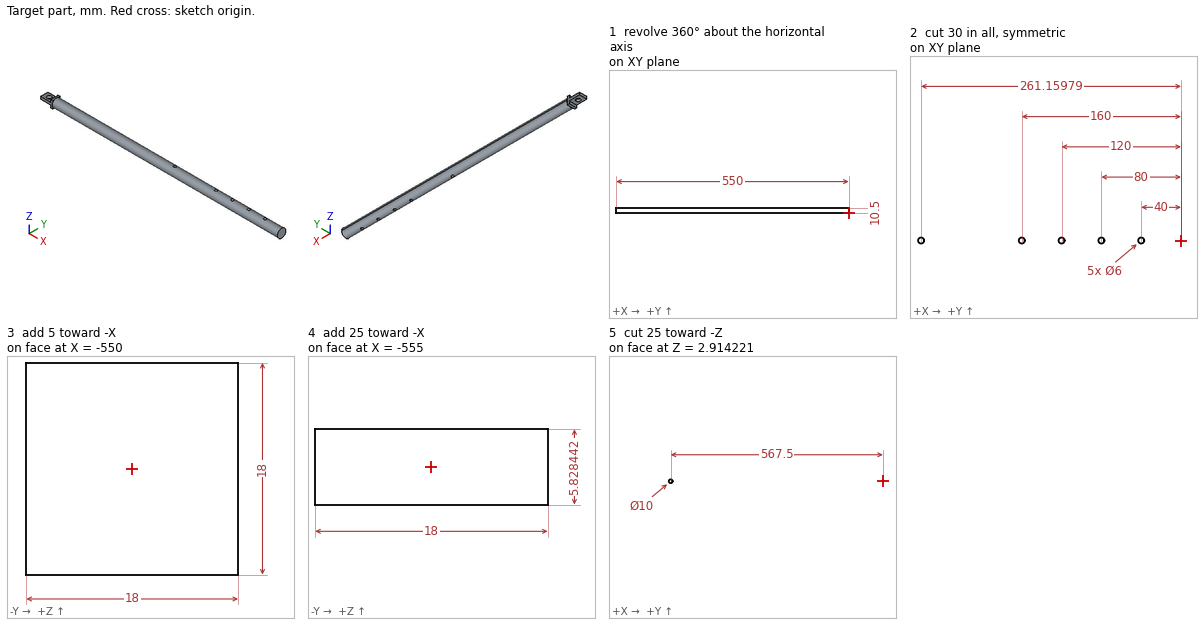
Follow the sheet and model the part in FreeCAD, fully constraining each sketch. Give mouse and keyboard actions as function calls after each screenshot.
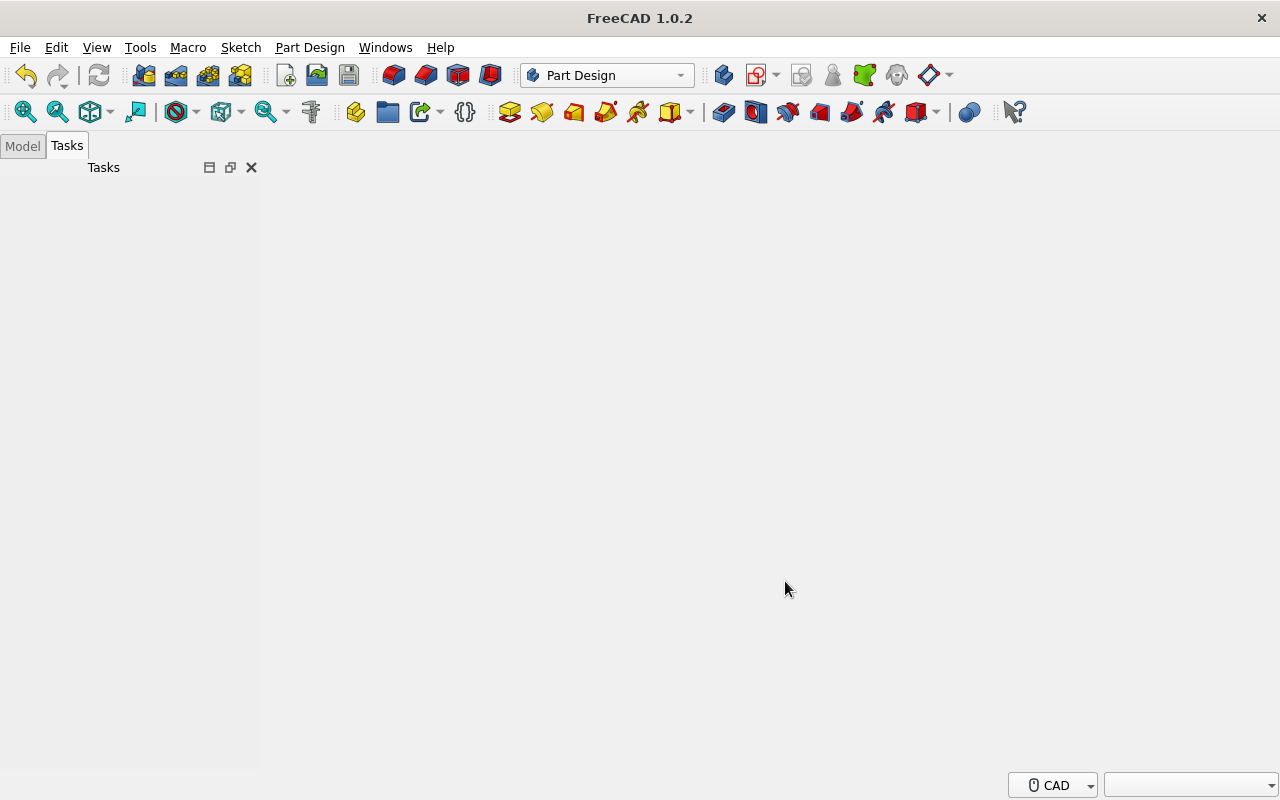
click(286, 76)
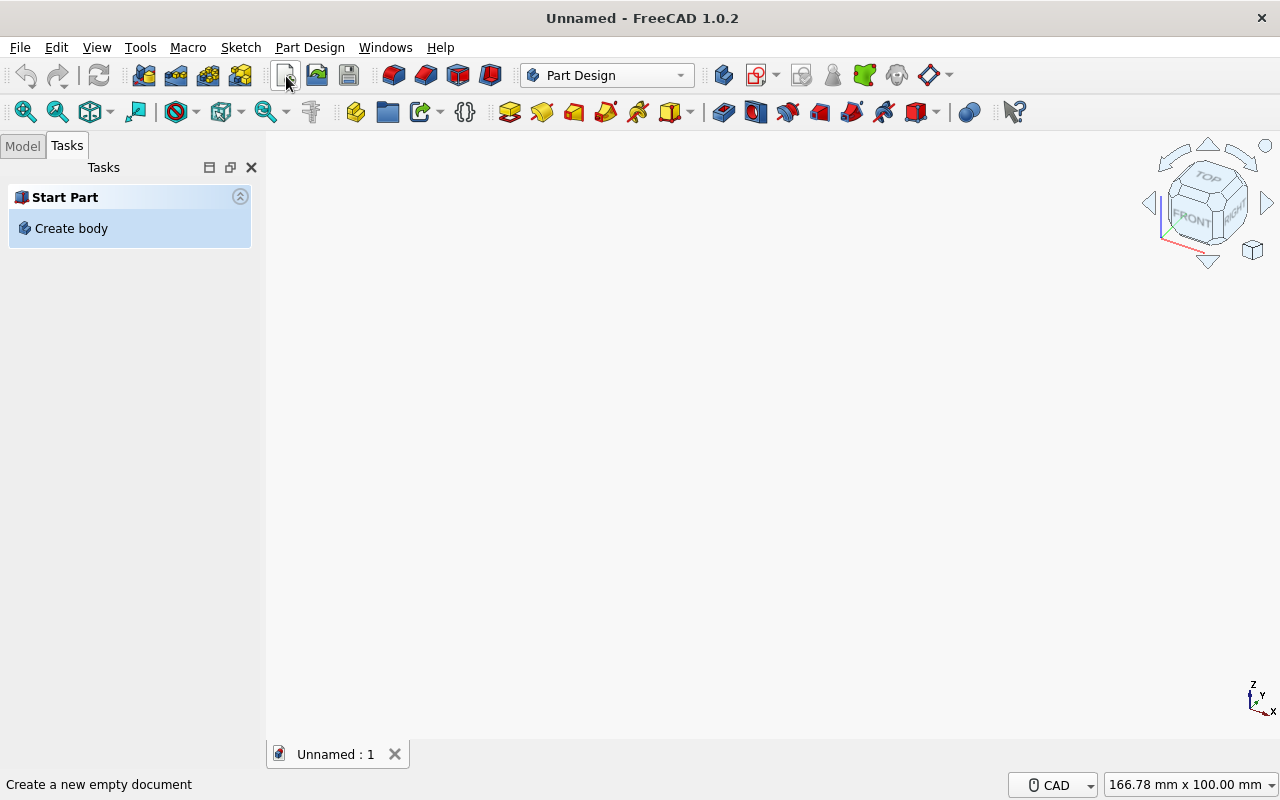
click(756, 76)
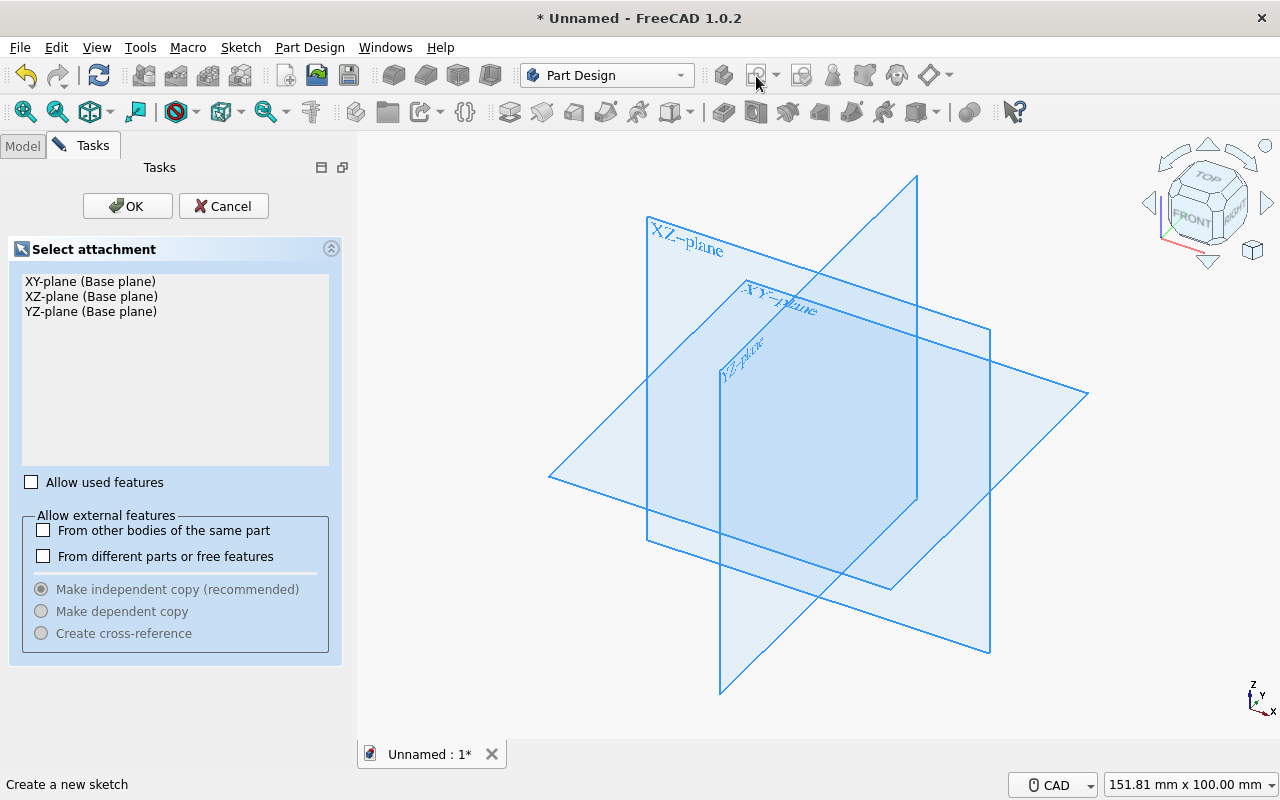
click(82, 282)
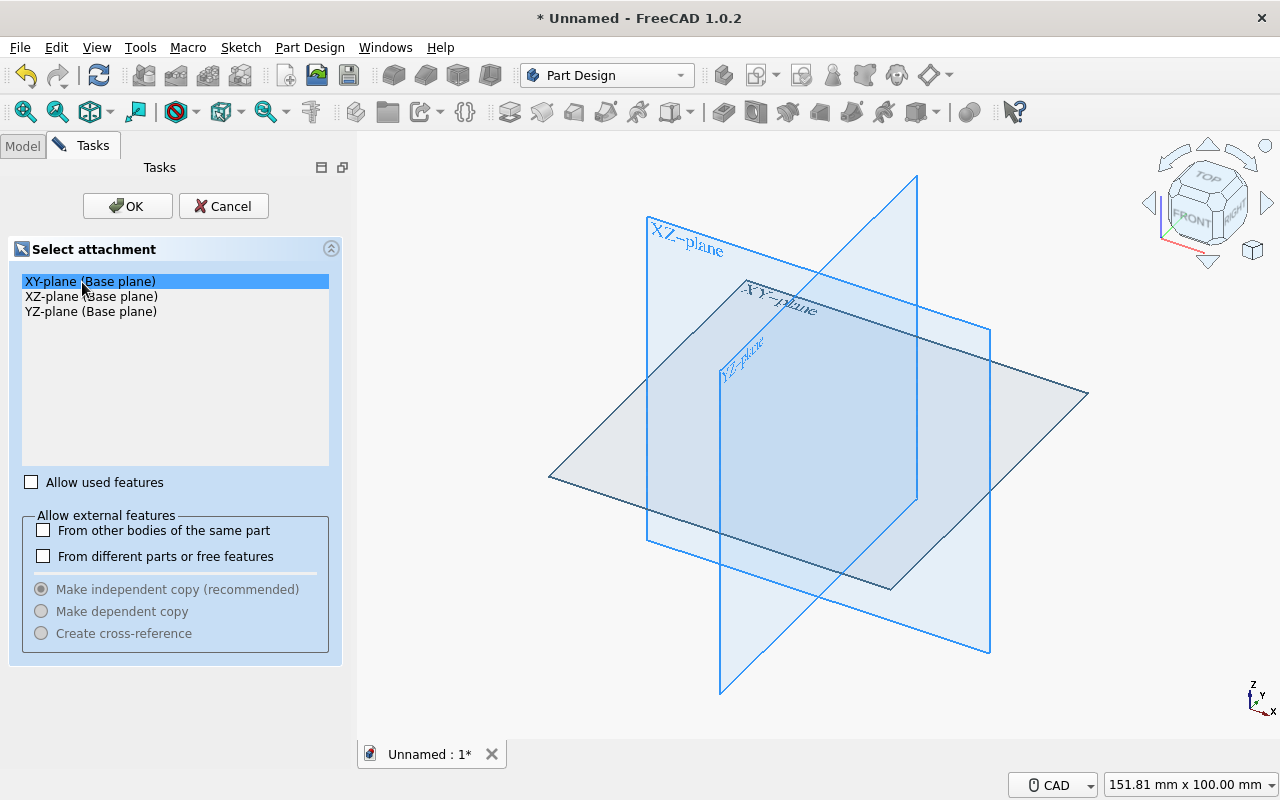
click(128, 206)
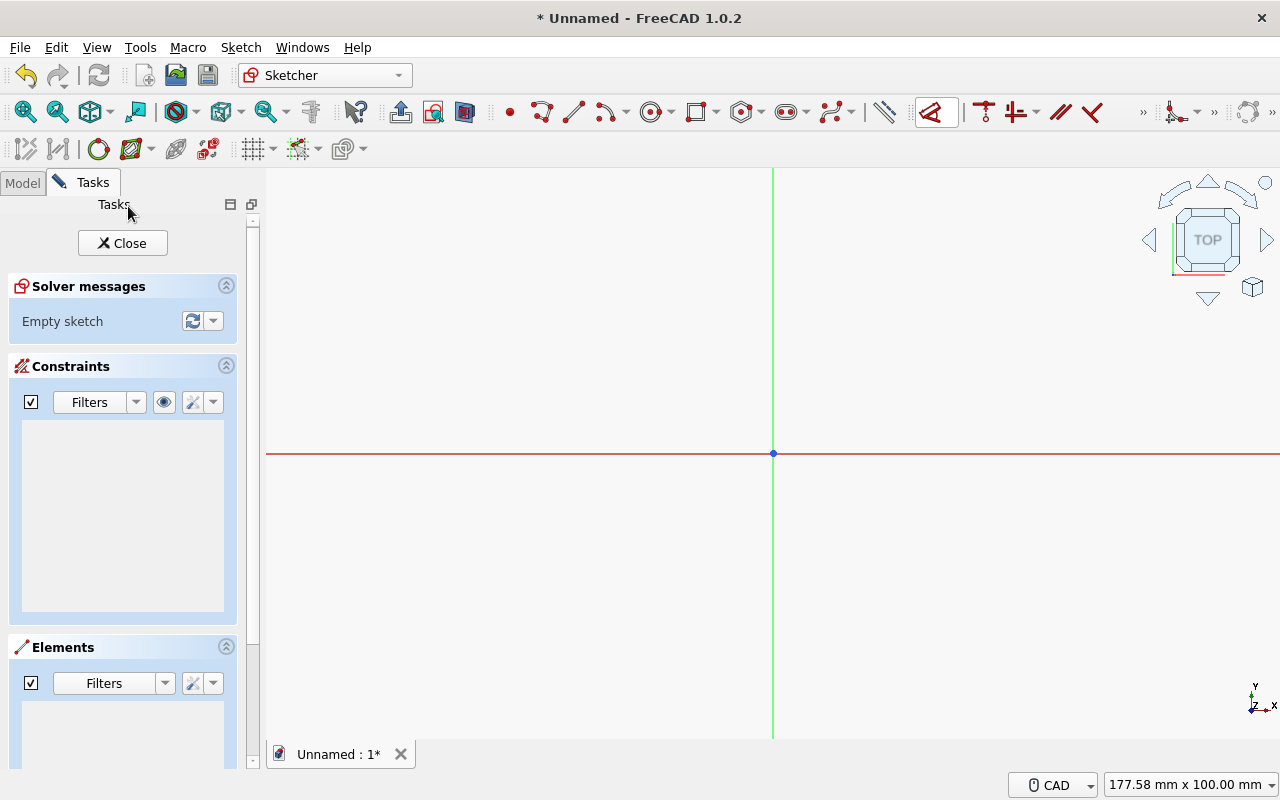
scroll(1084, 461, down, 8)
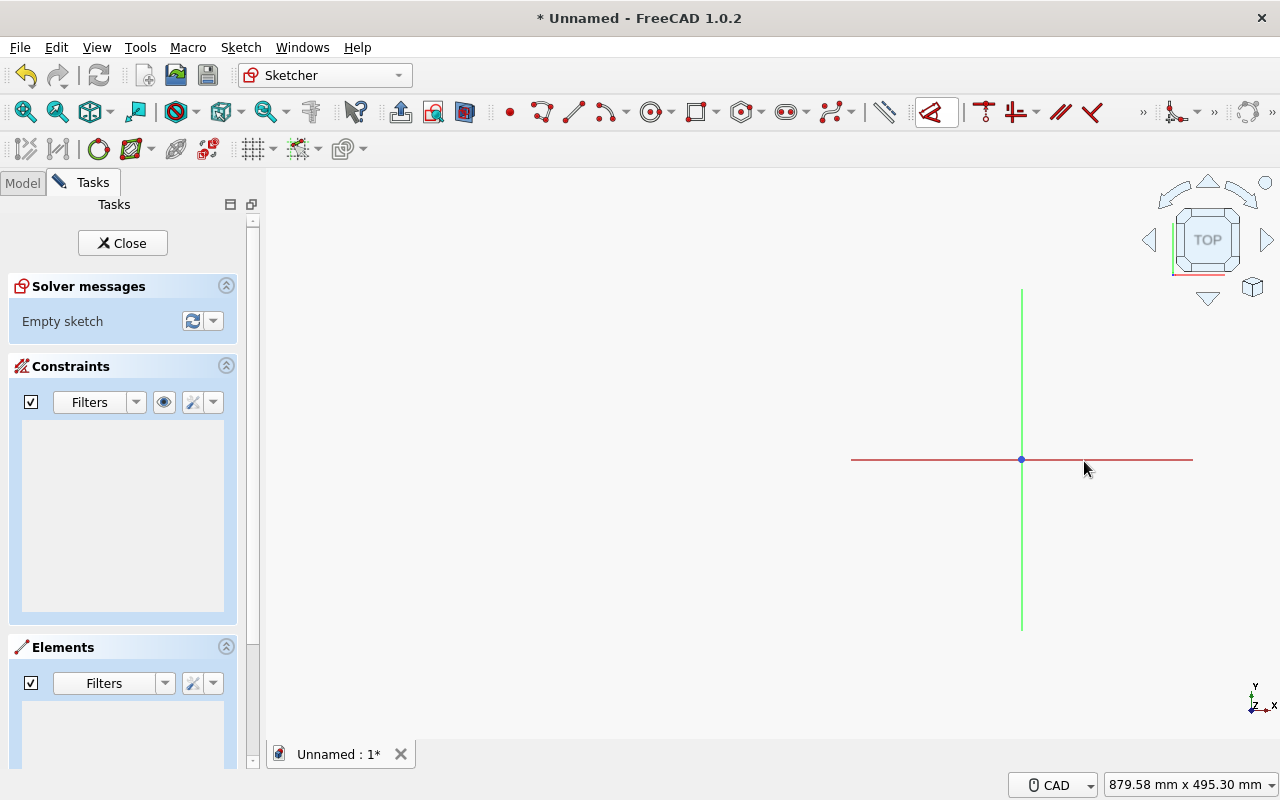
click(696, 112)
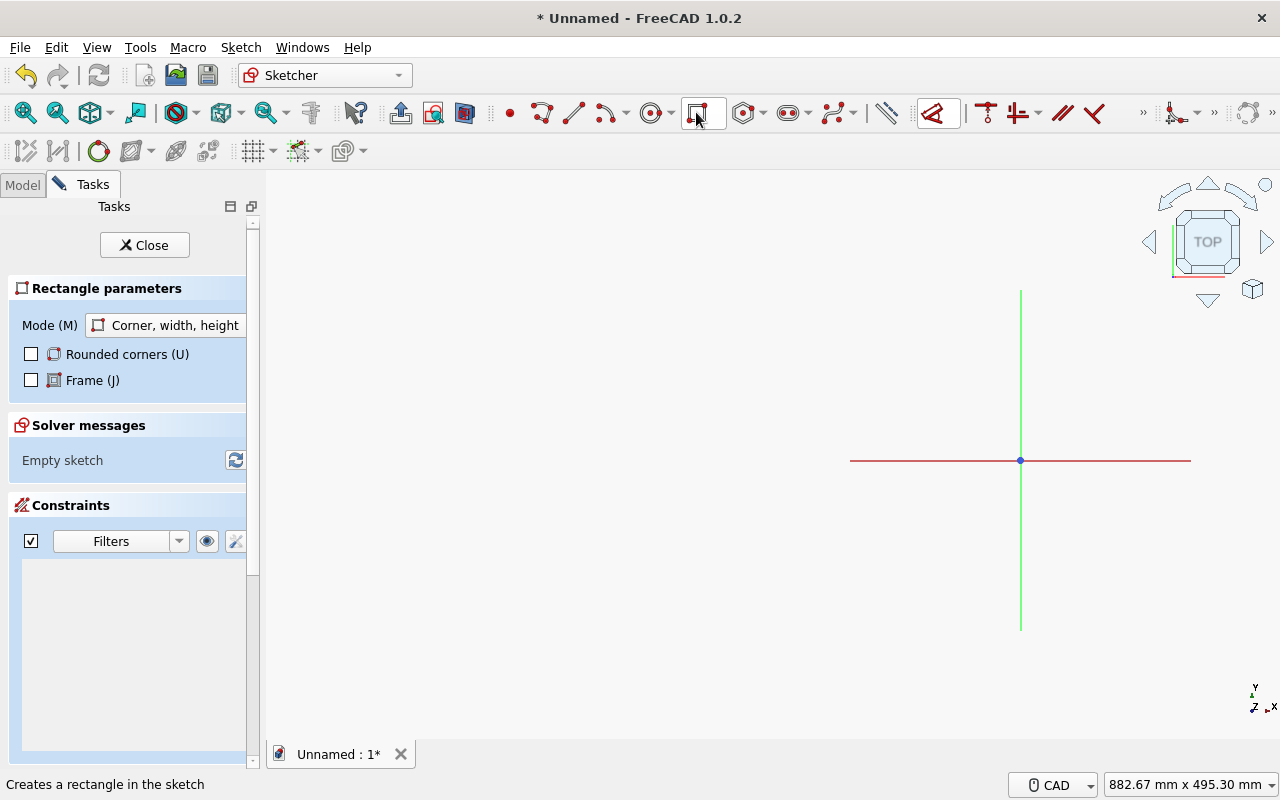
scroll(1021, 461, up, 2)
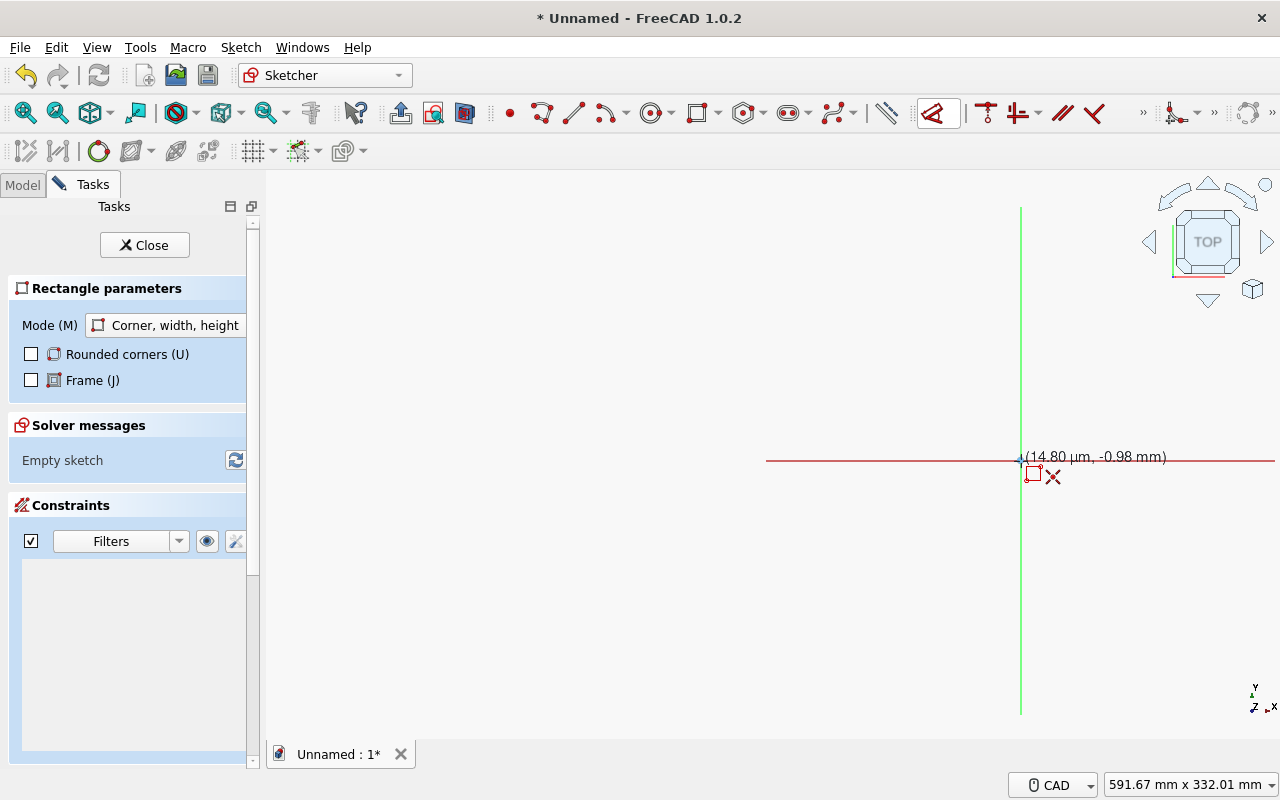
click(1021, 461)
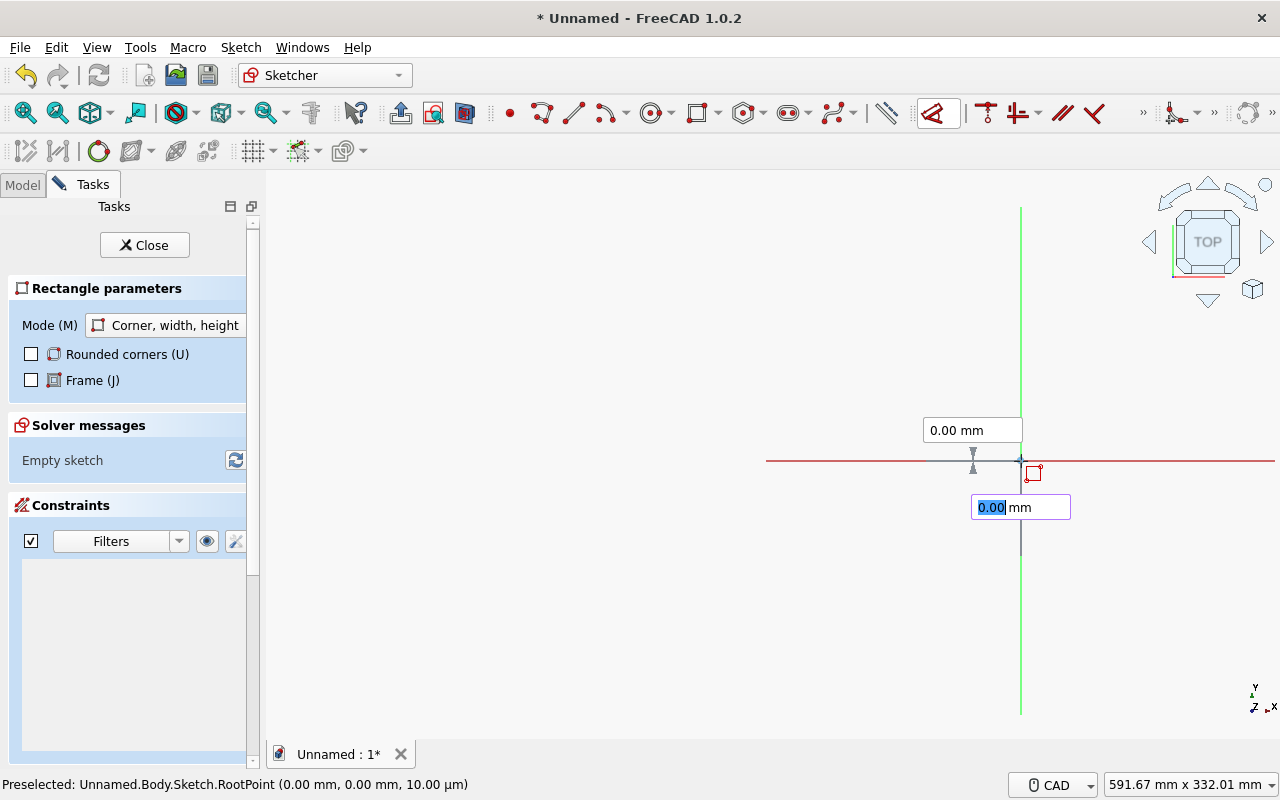
scroll(1020, 460, down, 2)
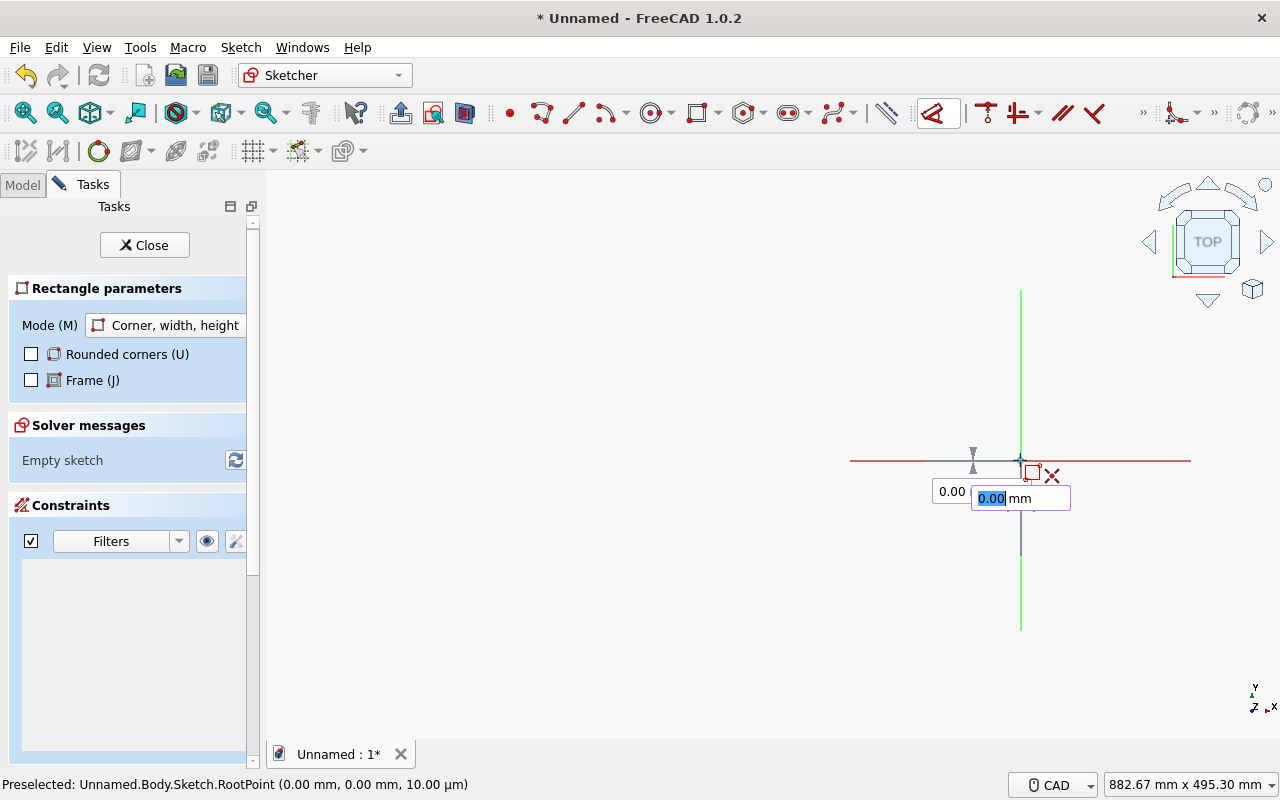
scroll(389, 448, up, 2)